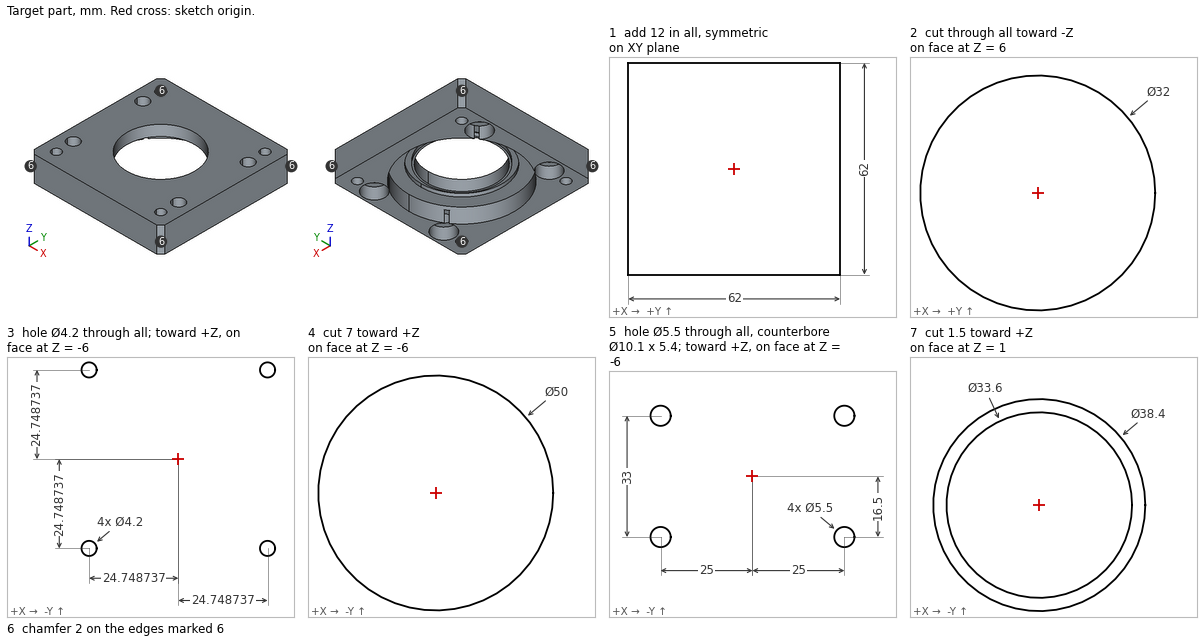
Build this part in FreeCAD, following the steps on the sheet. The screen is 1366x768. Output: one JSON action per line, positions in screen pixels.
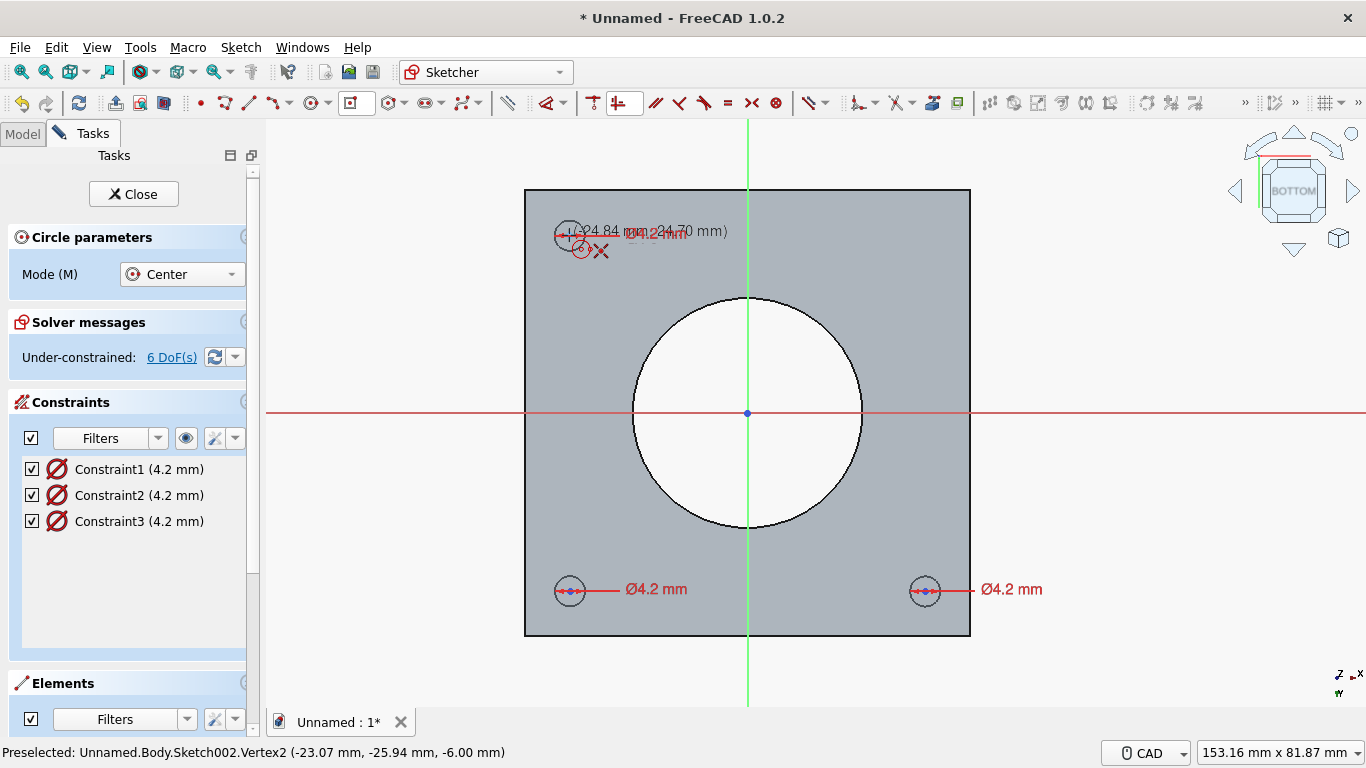
{"action": "scroll", "coordinate": [925, 235], "scroll_direction": "up", "scroll_amount": 3}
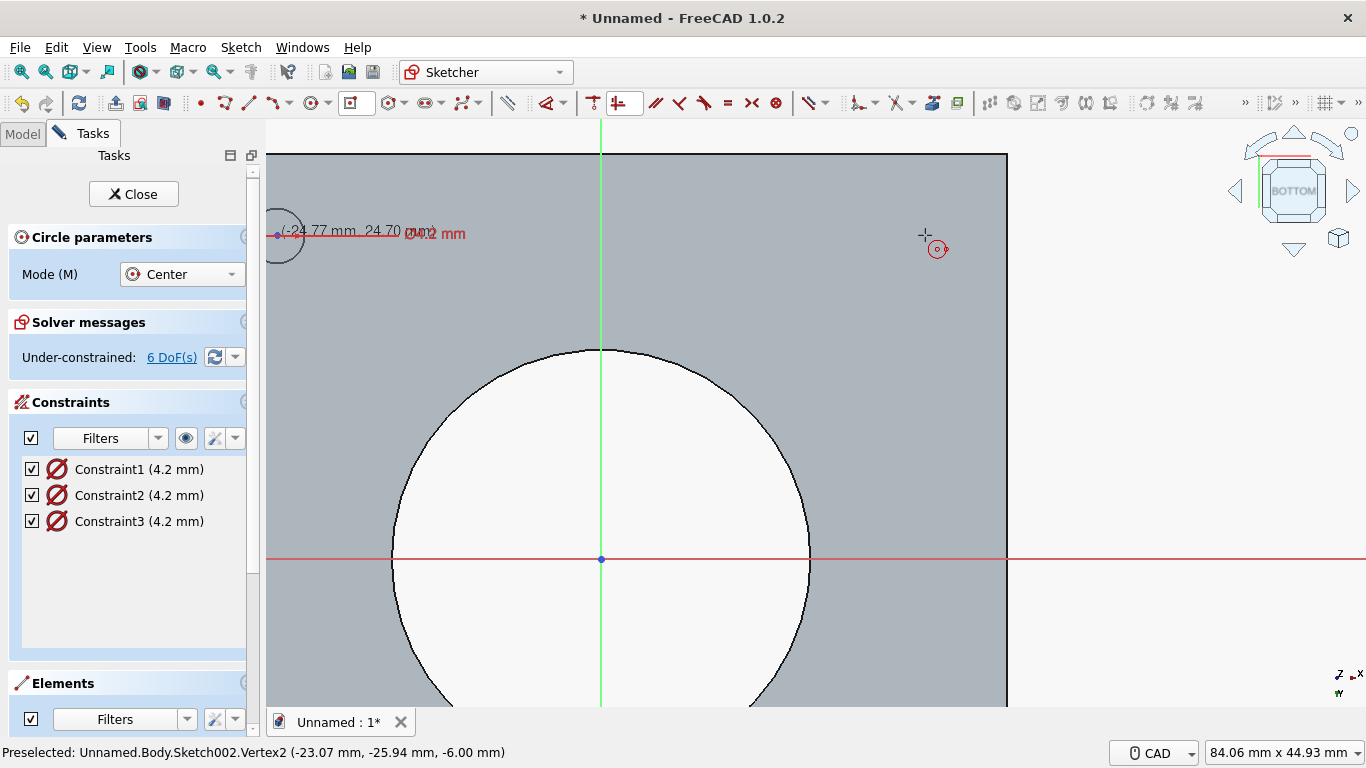
{"action": "left_click", "coordinate": [925, 235]}
{"action": "mouse_move", "coordinate": [944, 216]}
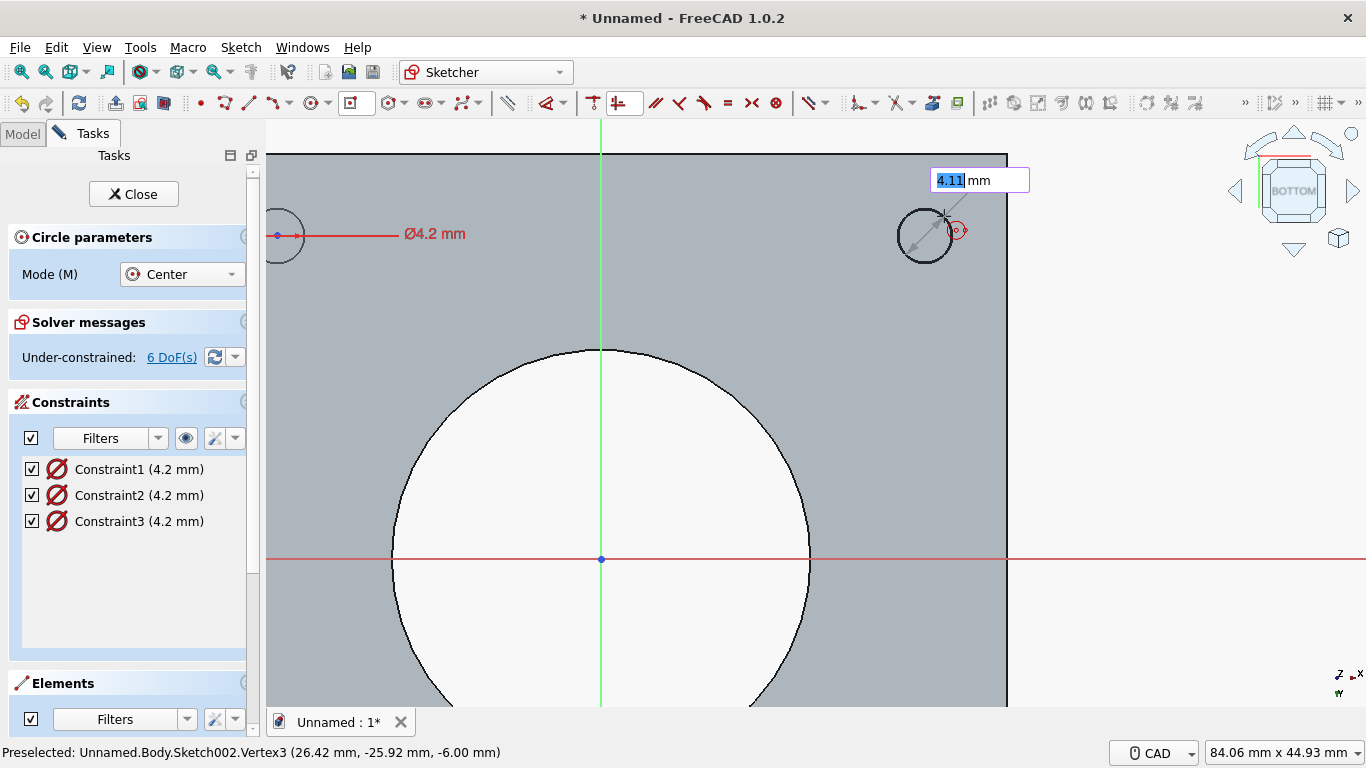
{"action": "type", "text": "4.2"}
{"action": "key", "text": "Return"}
{"action": "key", "text": "Escape"}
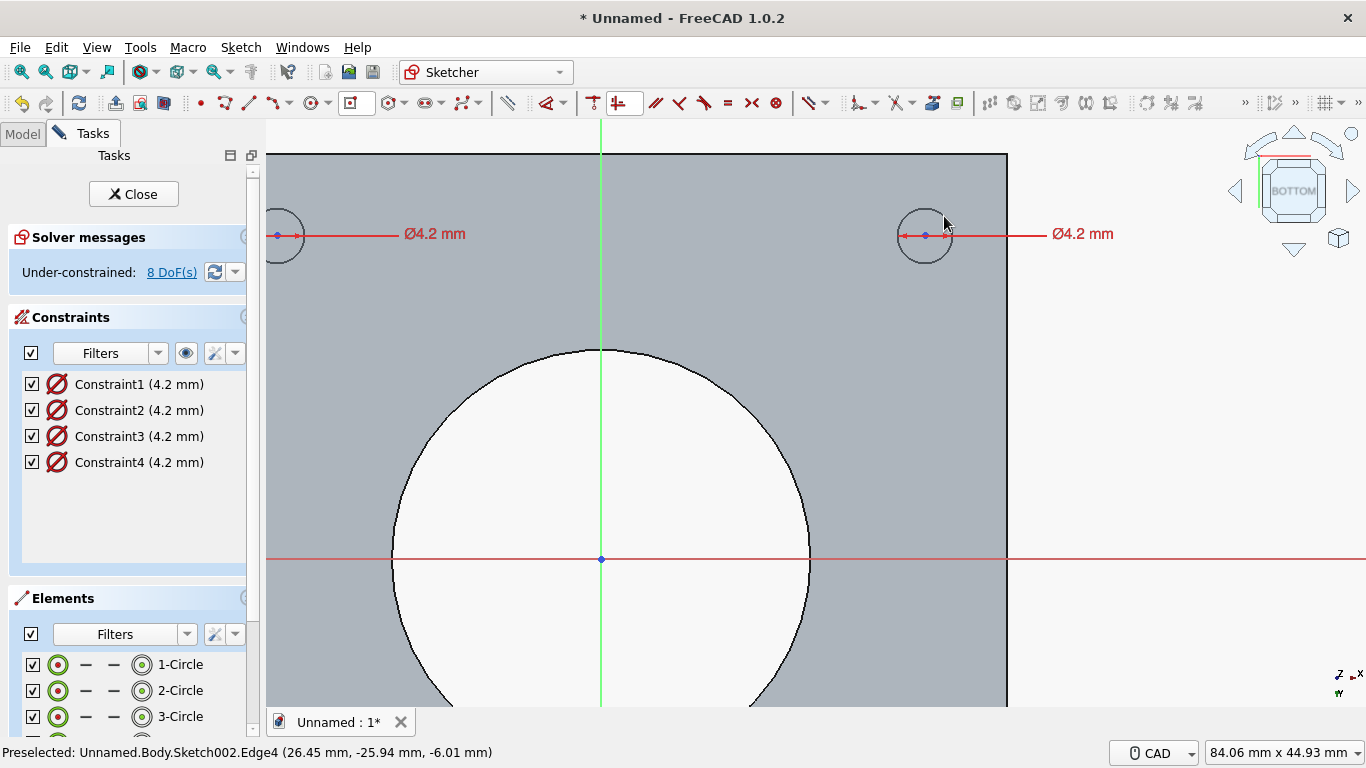
{"action": "scroll", "coordinate": [926, 235], "scroll_direction": "down", "scroll_amount": 3}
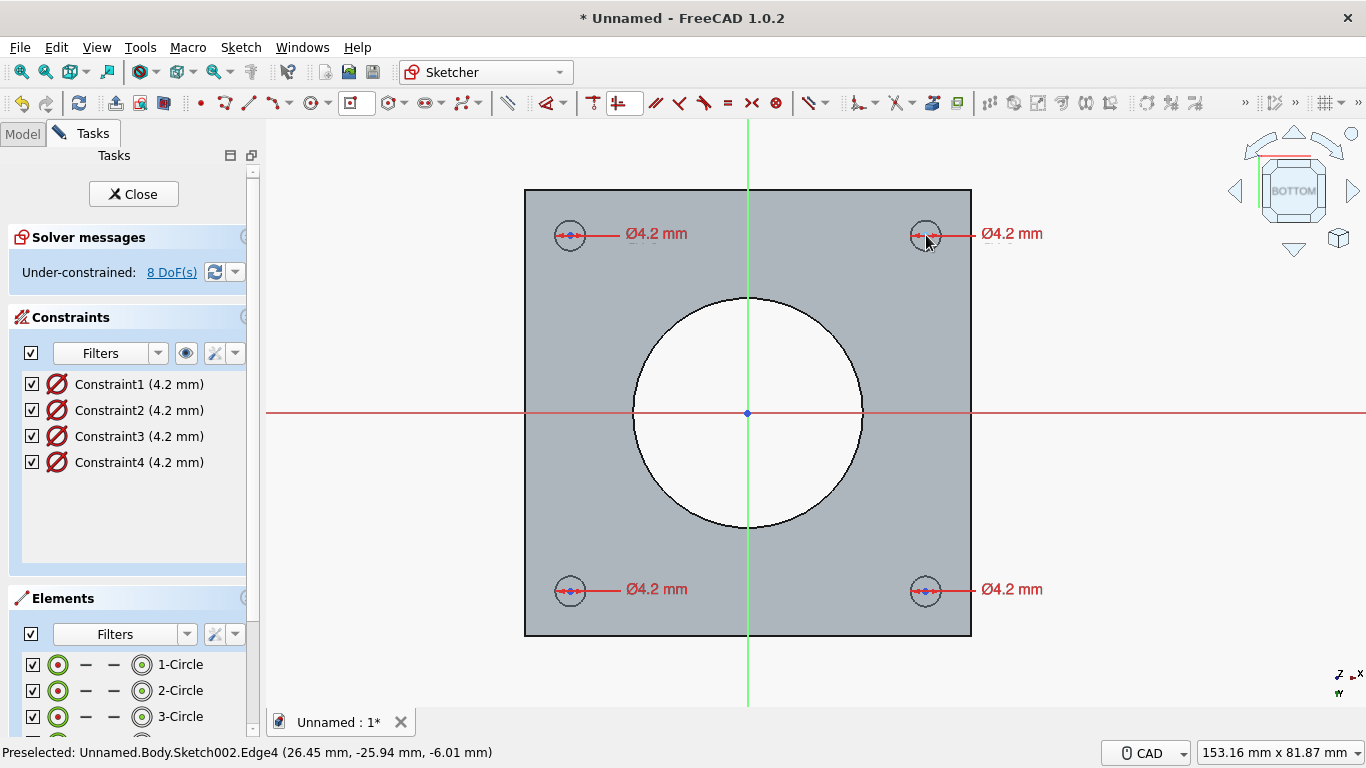
{"action": "left_click", "coordinate": [570, 591]}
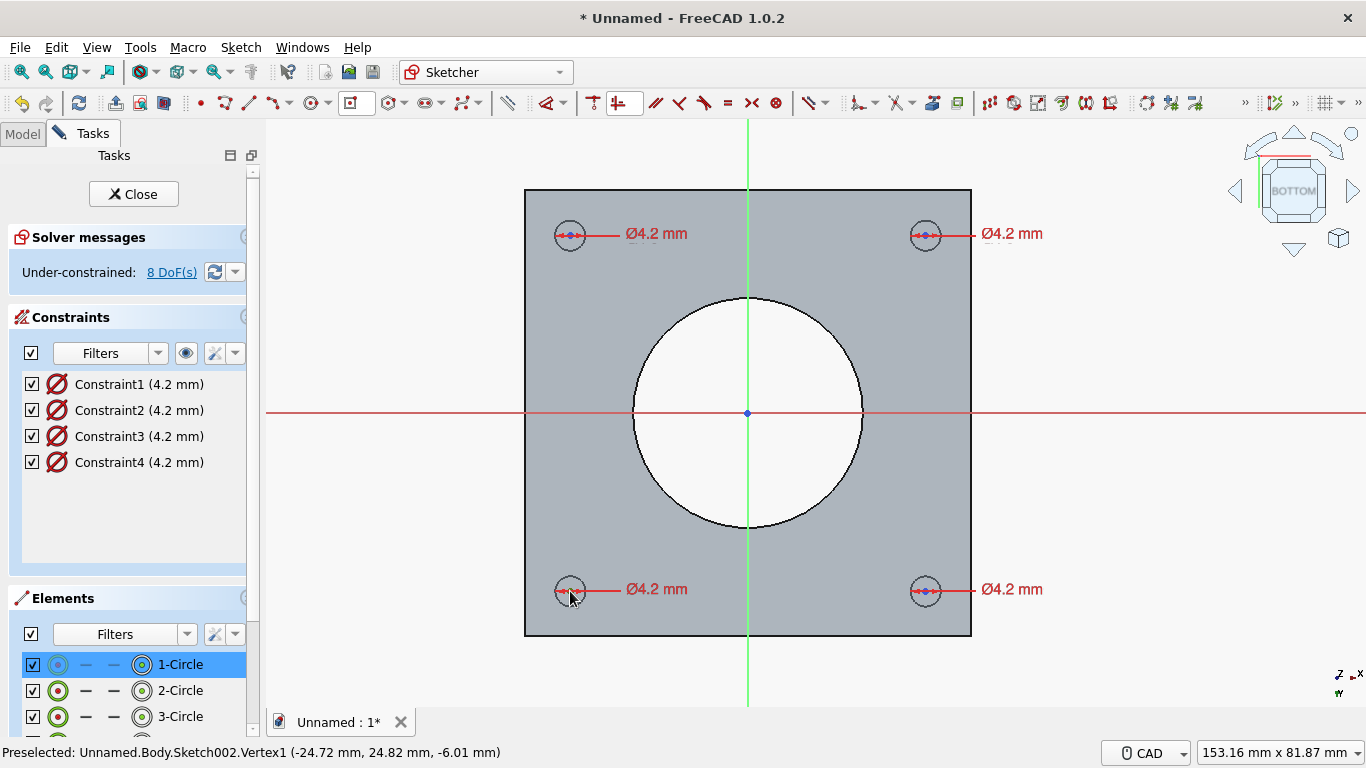
{"action": "left_click", "coordinate": [926, 591]}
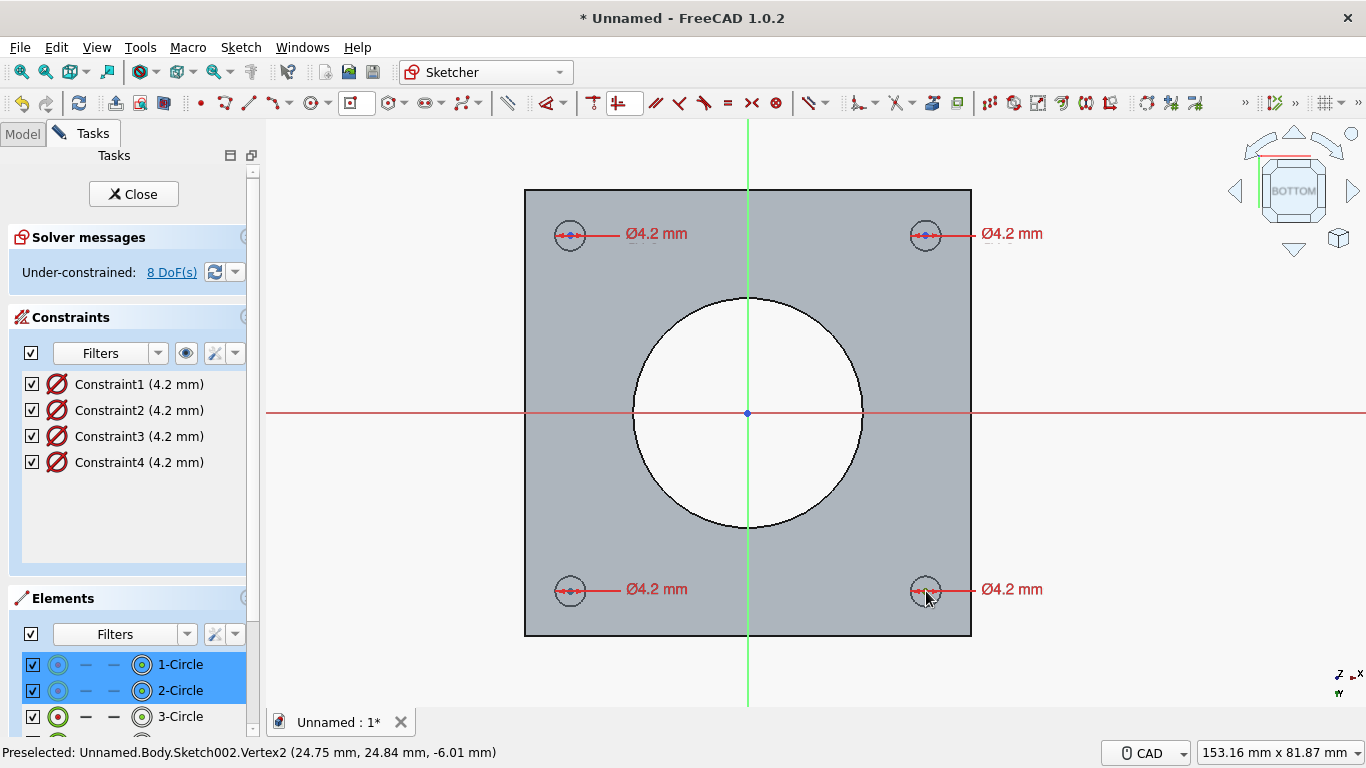
{"action": "left_click", "coordinate": [638, 104]}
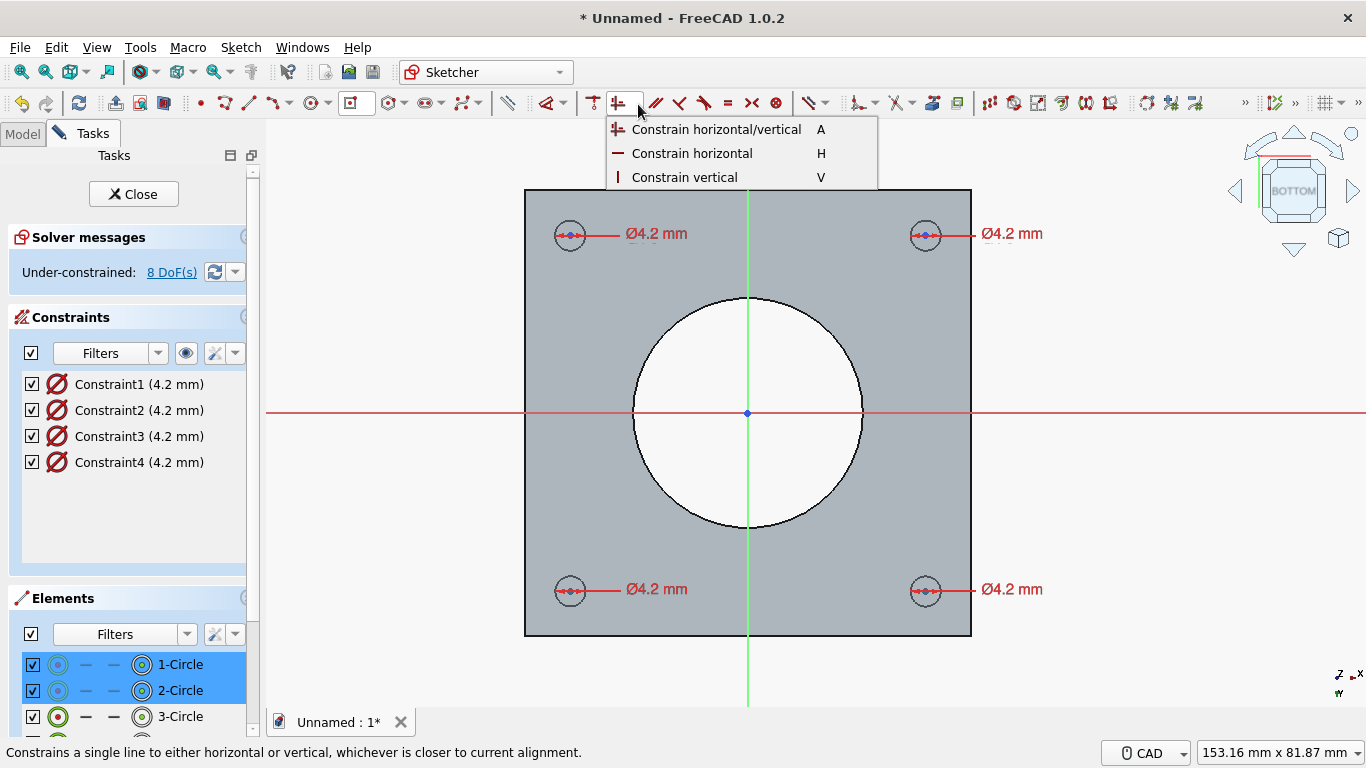
{"action": "left_click", "coordinate": [742, 153]}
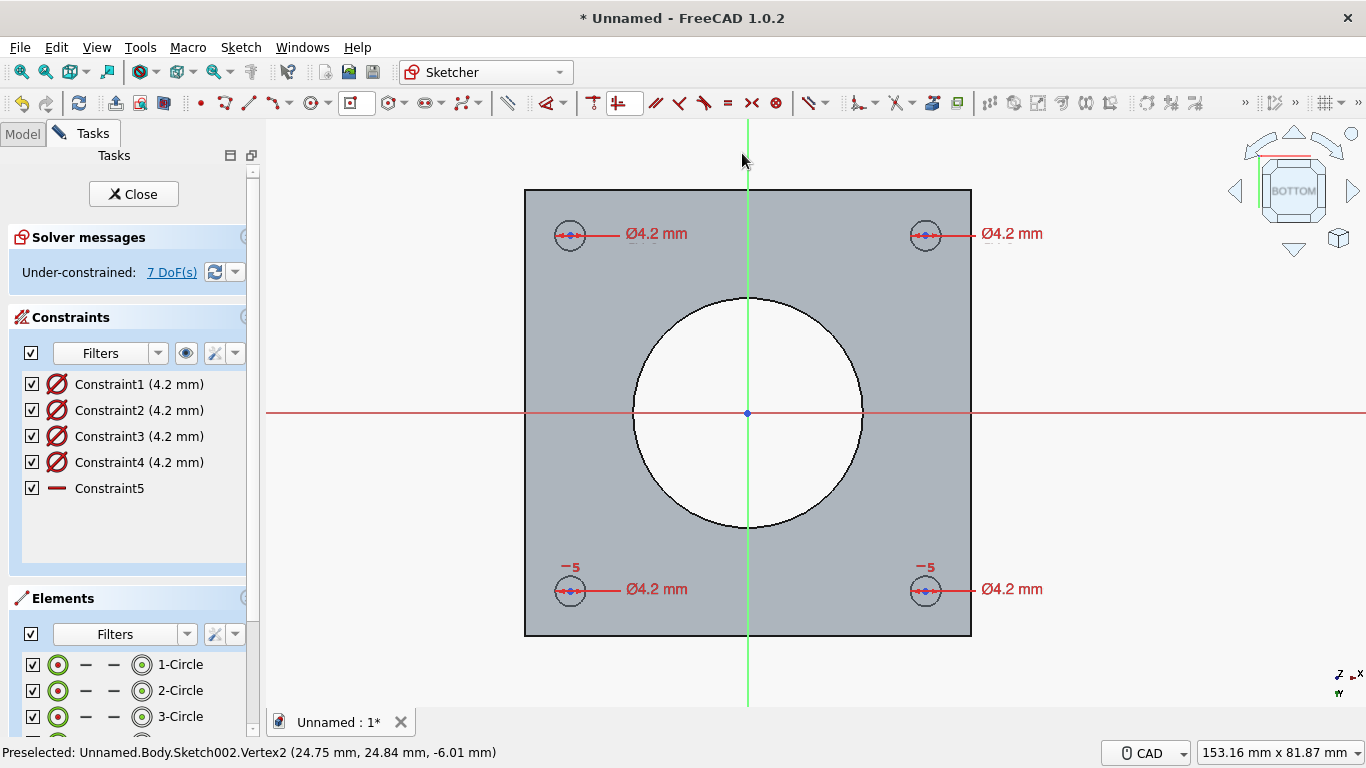
{"action": "left_click", "coordinate": [570, 591]}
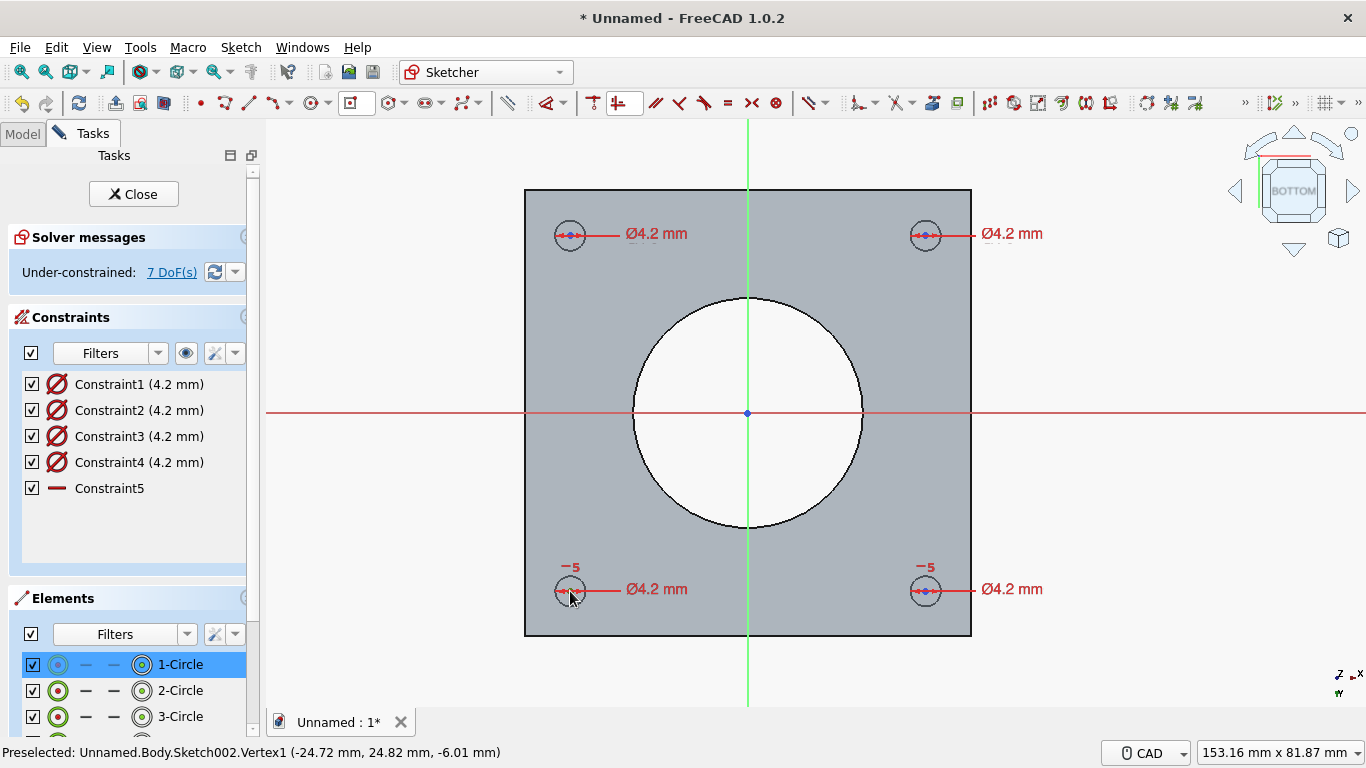
{"action": "left_click", "coordinate": [570, 236]}